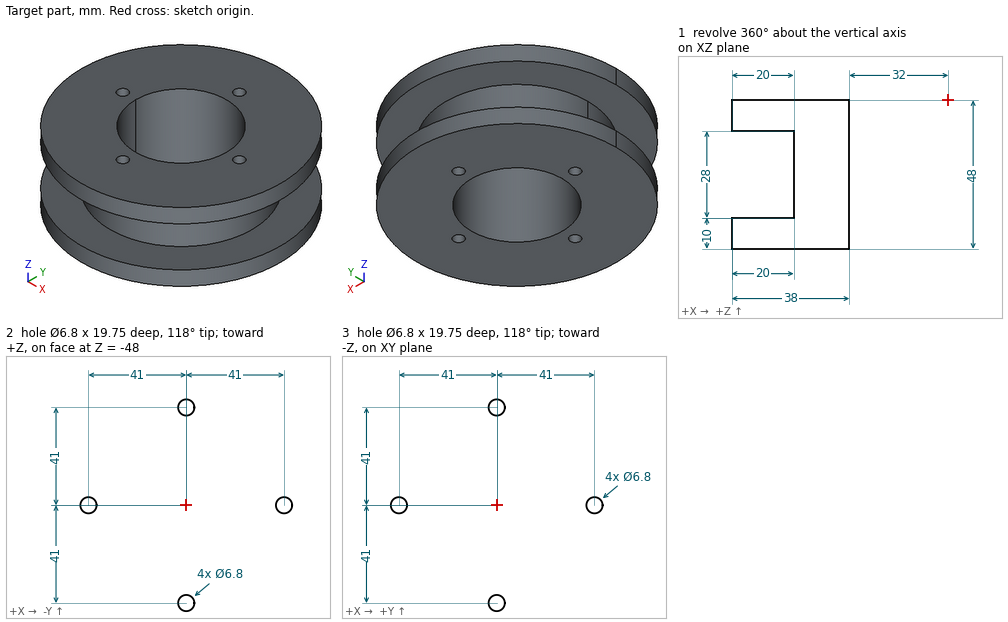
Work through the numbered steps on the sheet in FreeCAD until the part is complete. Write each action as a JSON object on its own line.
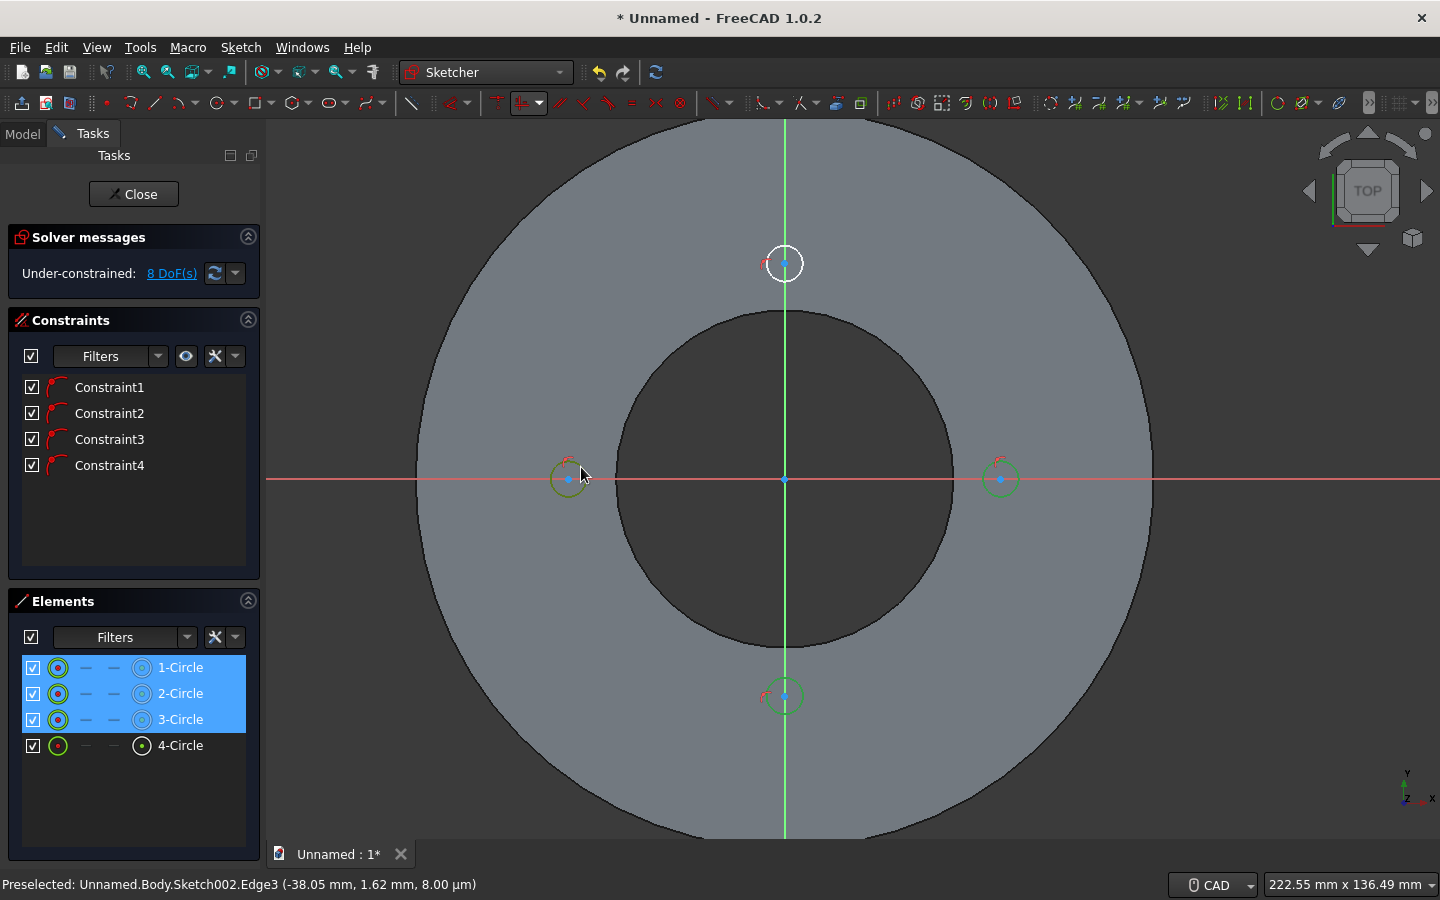
{"action": "left_click", "coordinate": [797, 251]}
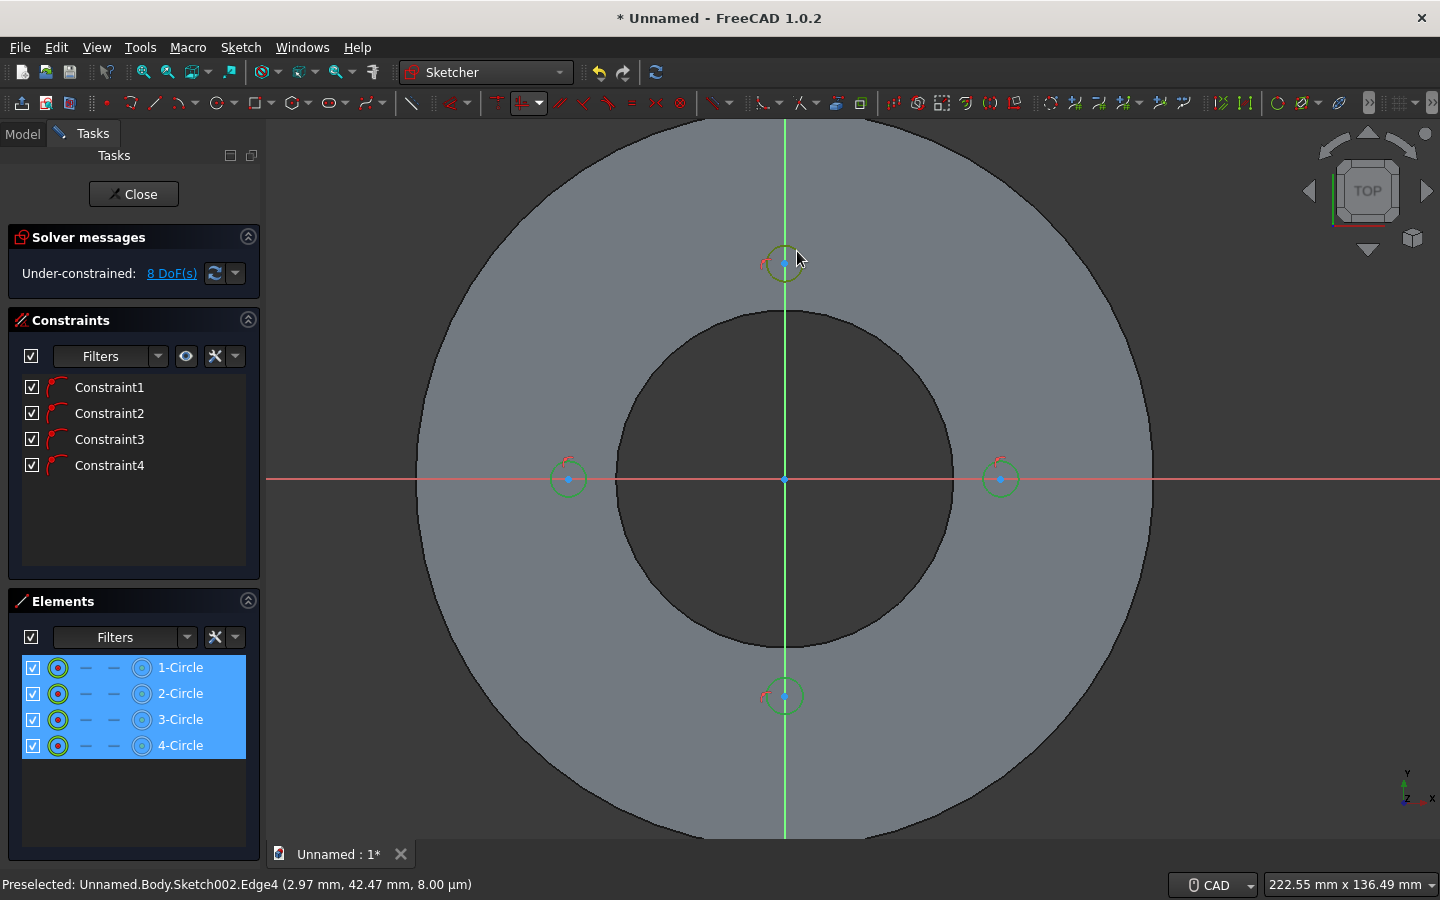
{"action": "left_click", "coordinate": [632, 104]}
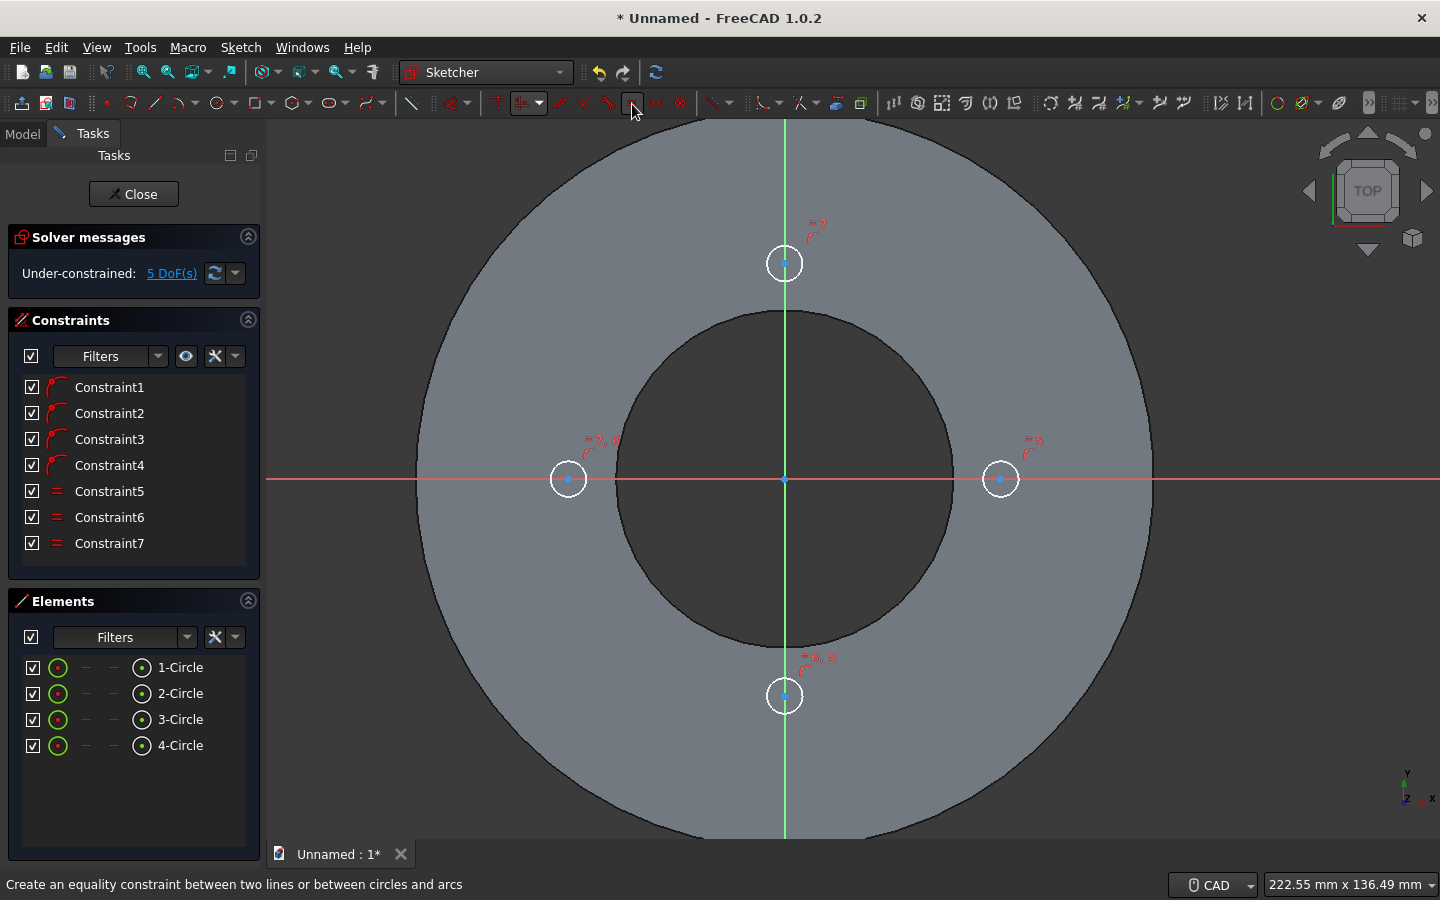
{"action": "left_click", "coordinate": [450, 104]}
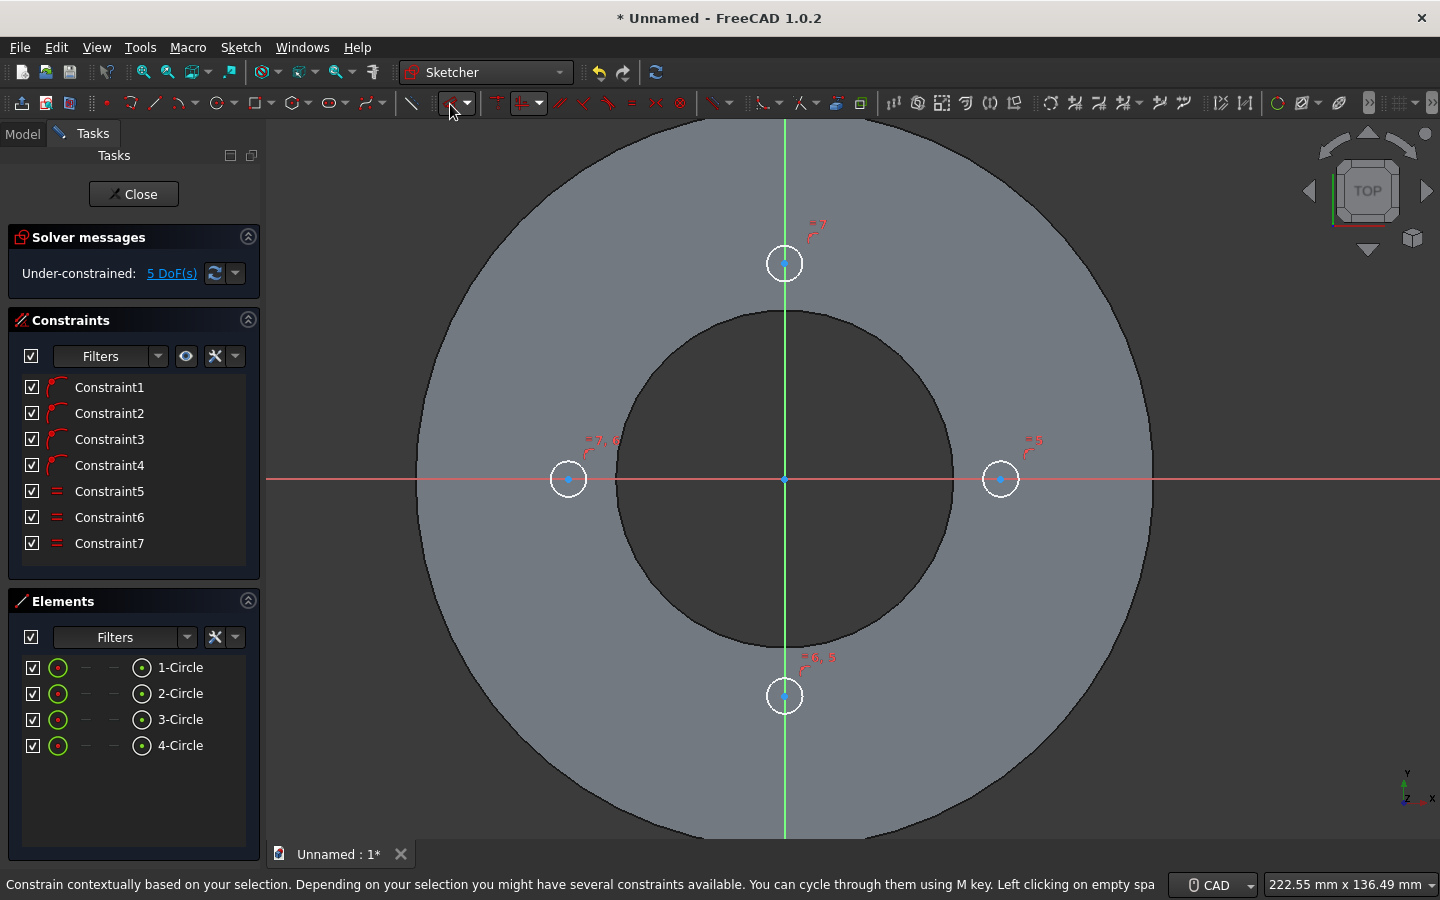
{"action": "left_click", "coordinate": [1013, 467]}
{"action": "left_click", "coordinate": [1036, 444]}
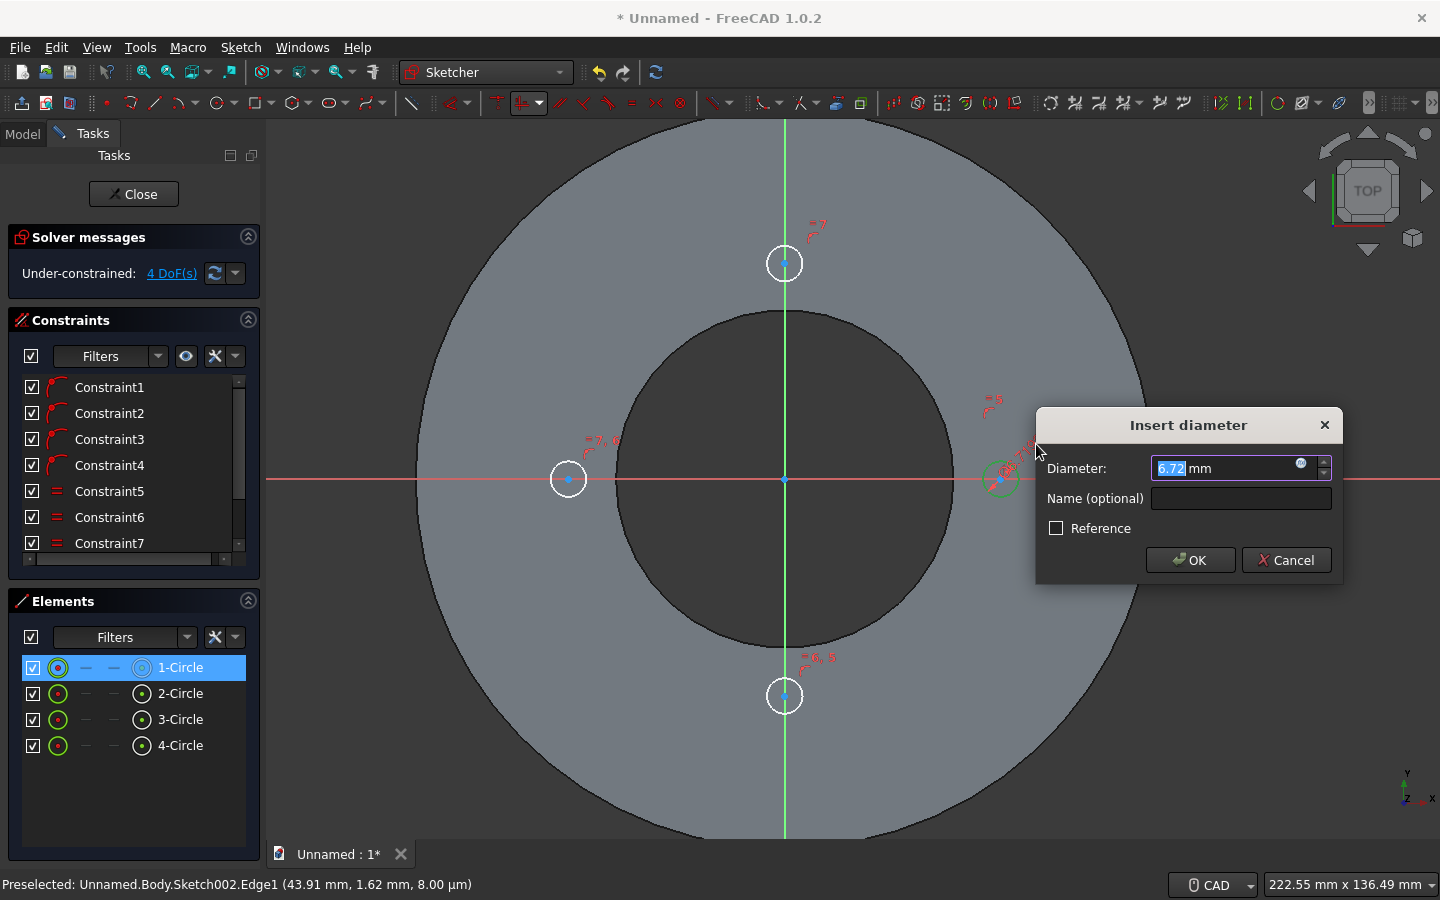
{"action": "type", "text": "6.8"}
{"action": "key", "text": "Return"}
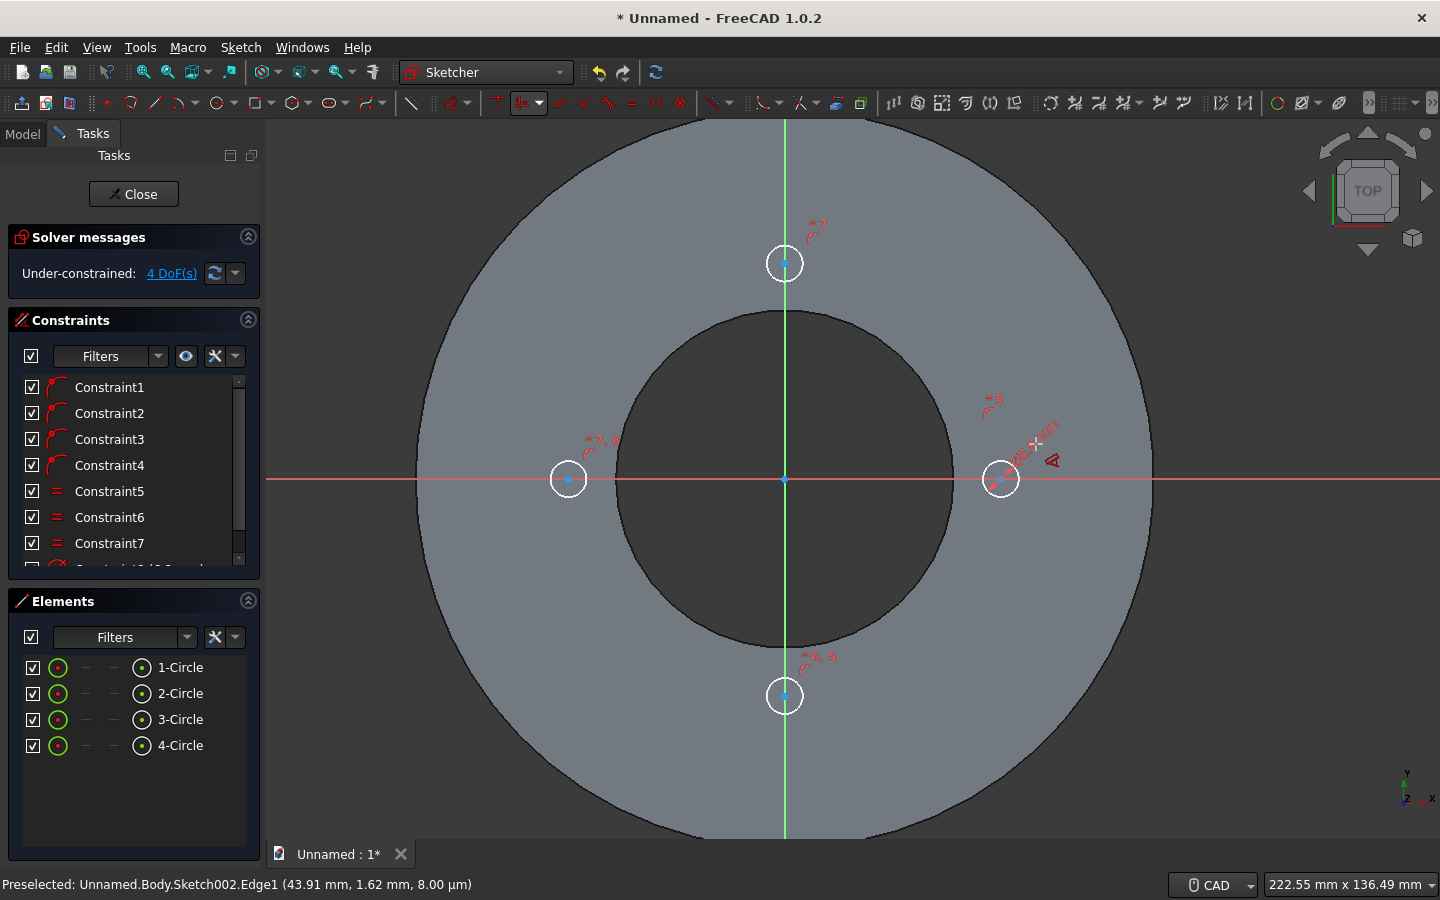
{"action": "left_click", "coordinate": [1001, 479]}
{"action": "left_click", "coordinate": [893, 513]}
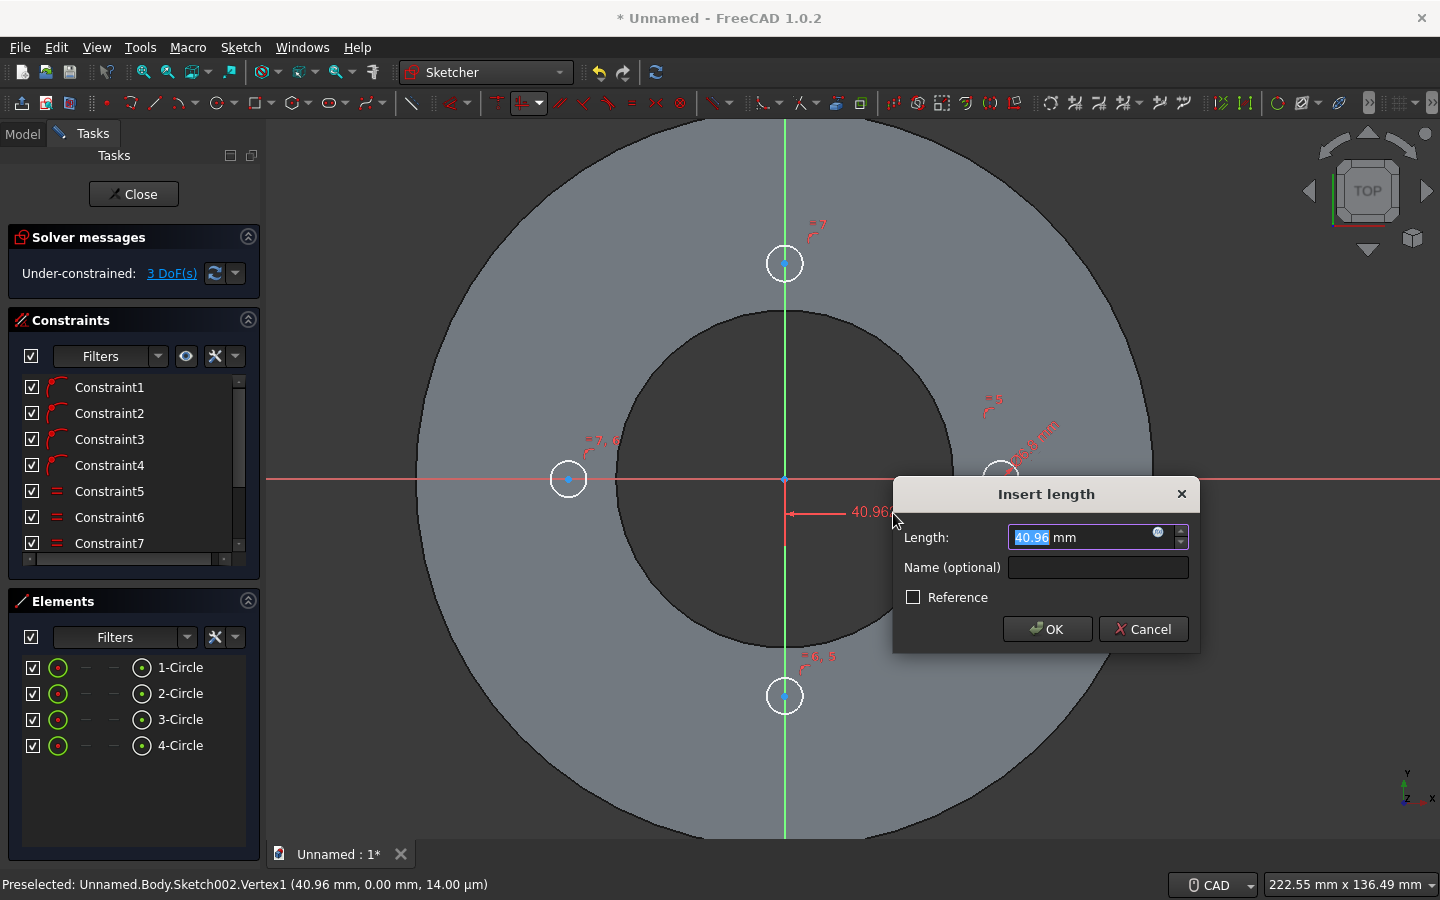
{"action": "type", "text": "41"}
{"action": "key", "text": "Return"}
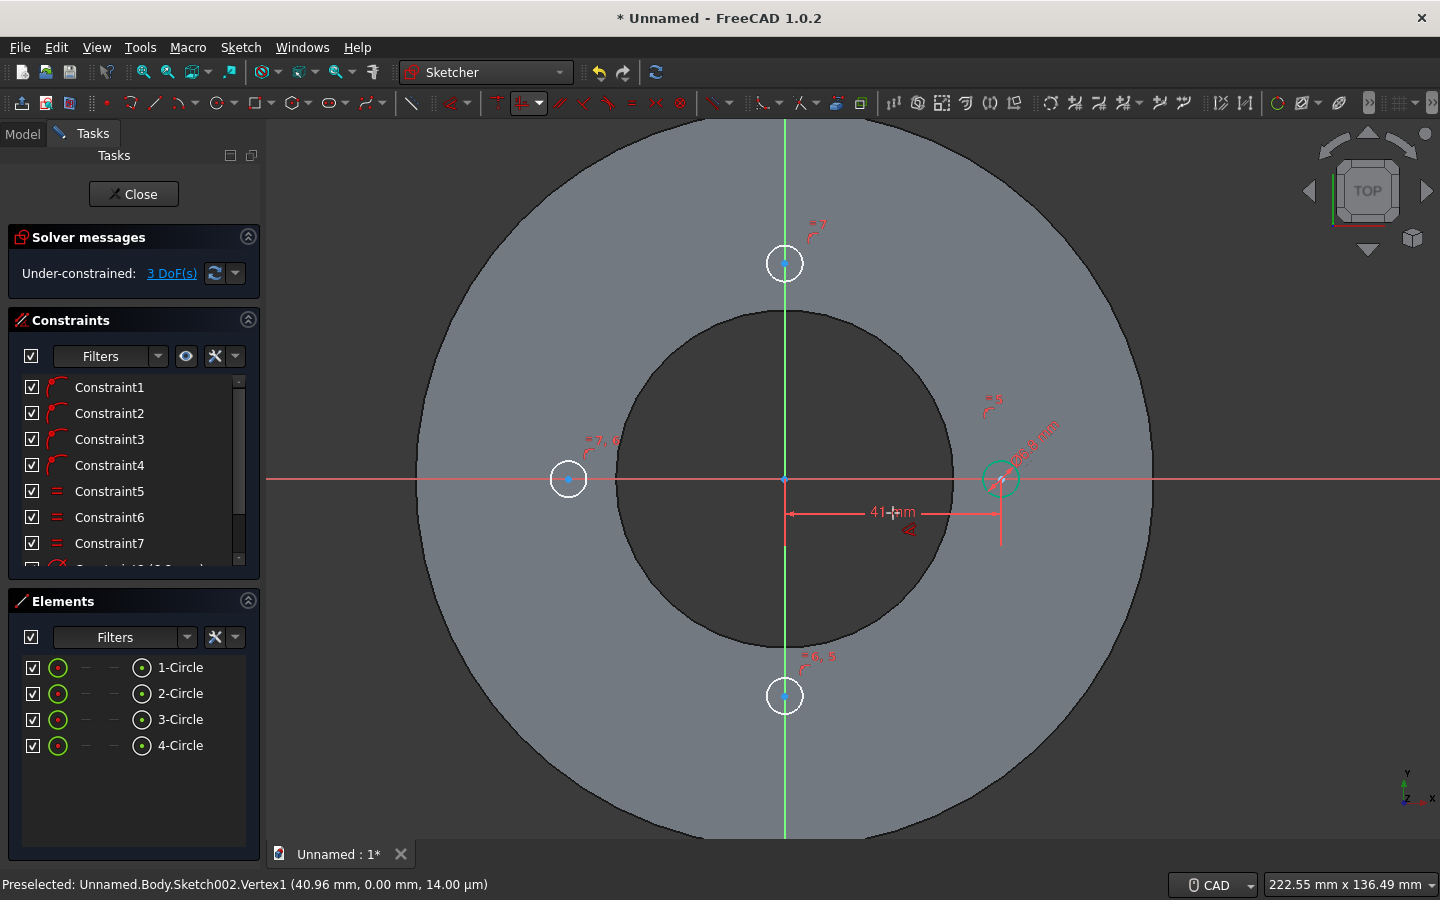
{"action": "left_click", "coordinate": [785, 696]}
{"action": "left_click", "coordinate": [819, 588]}